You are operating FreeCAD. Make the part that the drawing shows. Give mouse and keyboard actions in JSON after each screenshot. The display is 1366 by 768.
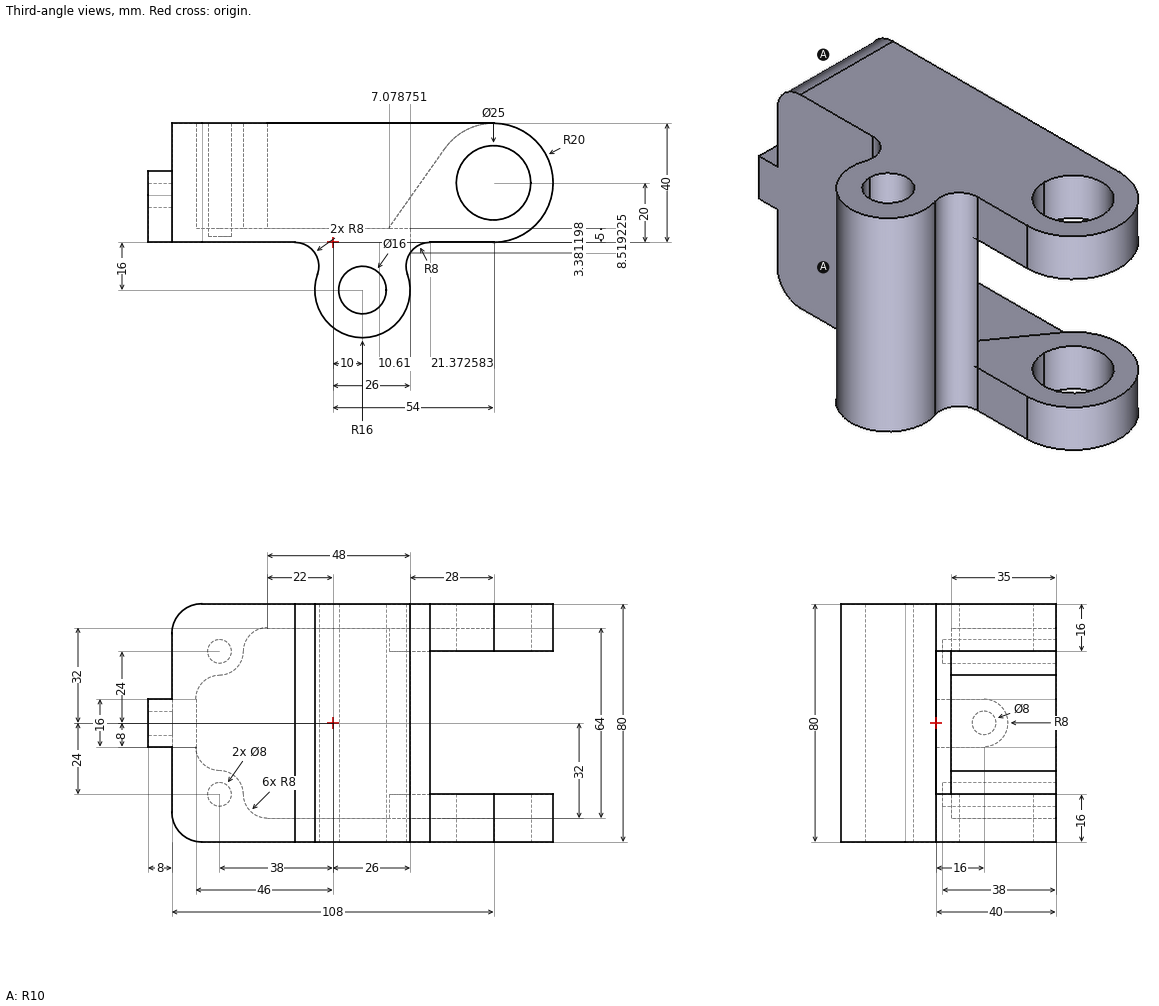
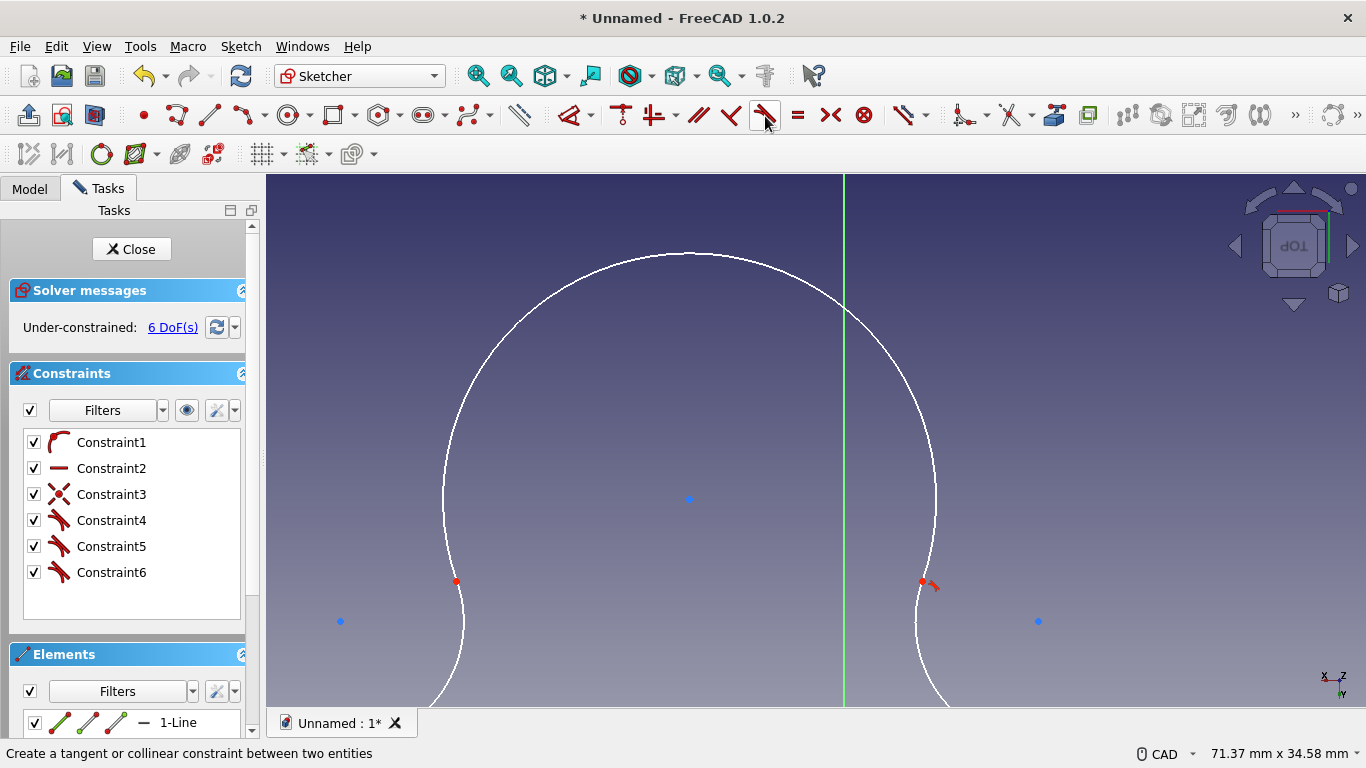
{"action": "left_click", "coordinate": [860, 322]}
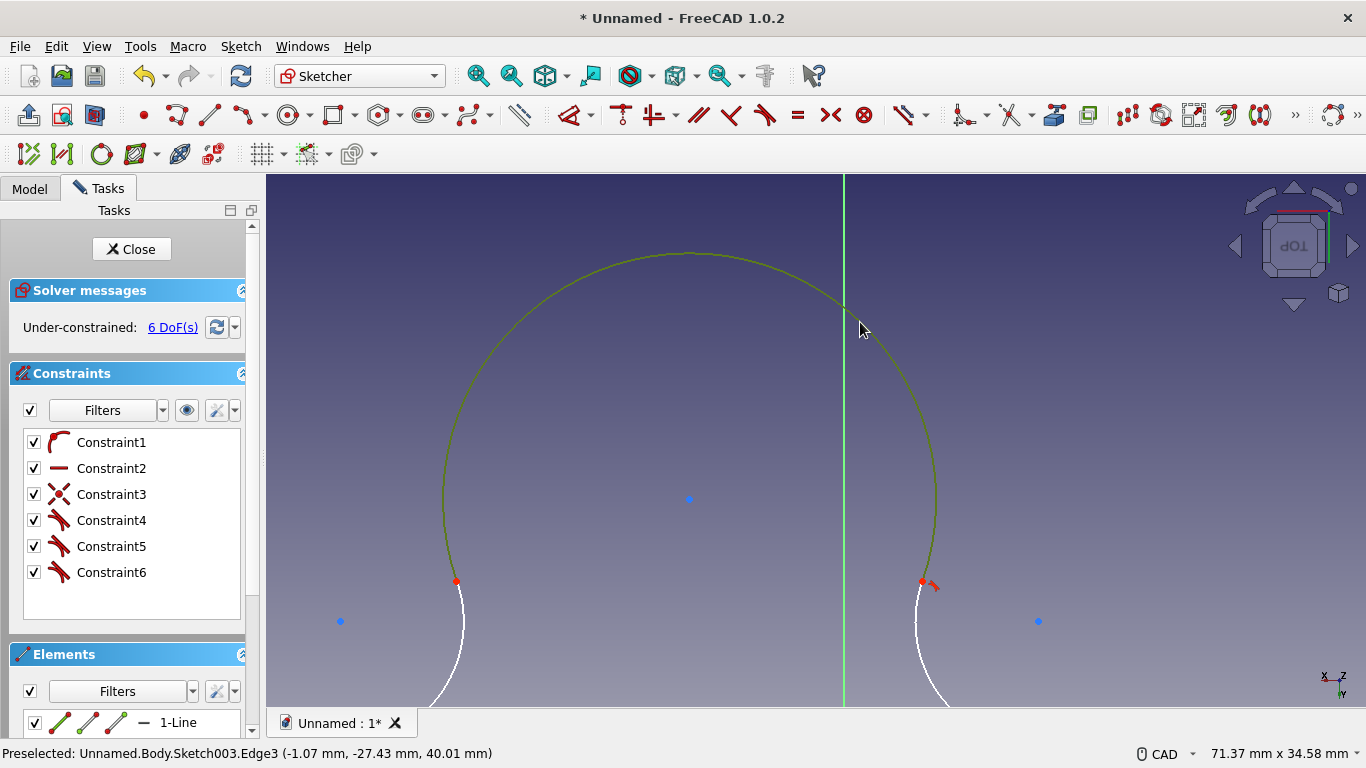
{"action": "left_click", "coordinate": [460, 651]}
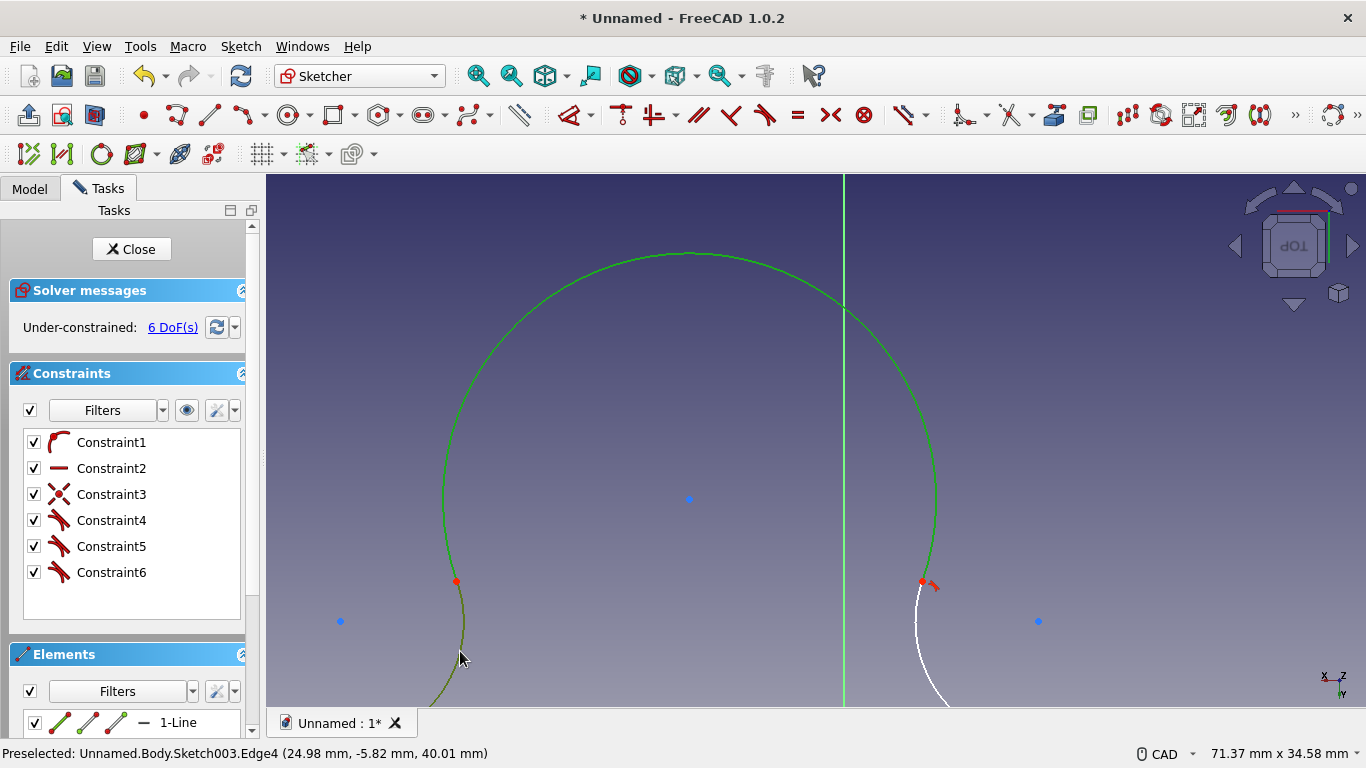
{"action": "left_click", "coordinate": [765, 116]}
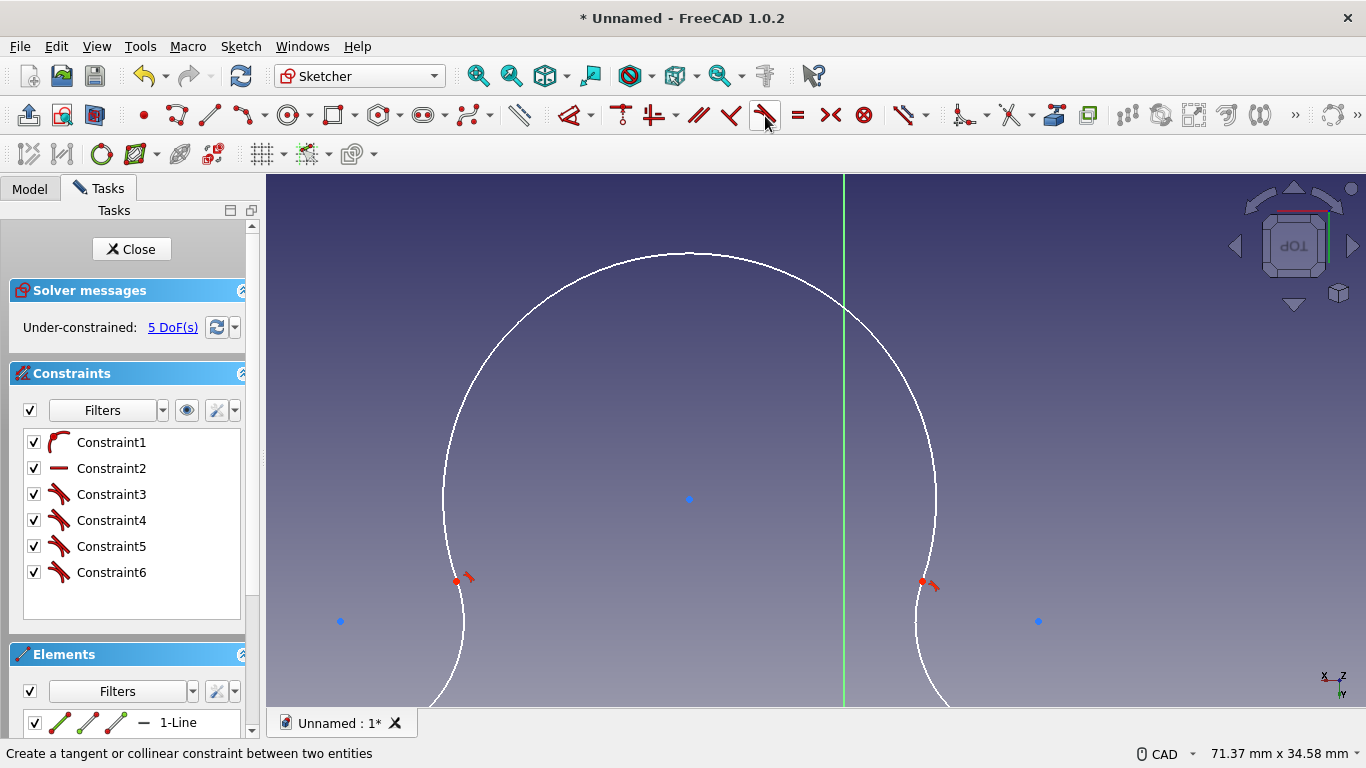
{"action": "left_click", "coordinate": [919, 651]}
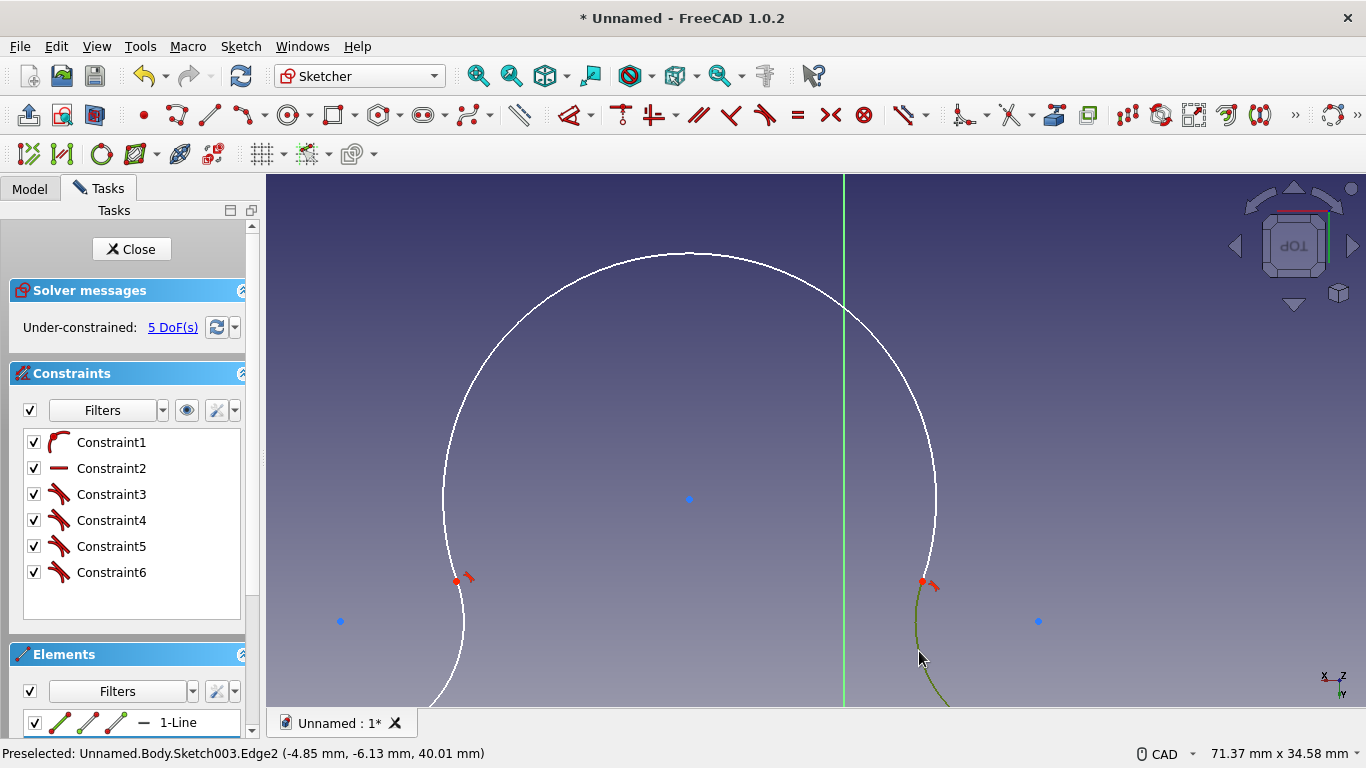
{"action": "left_click", "coordinate": [460, 651]}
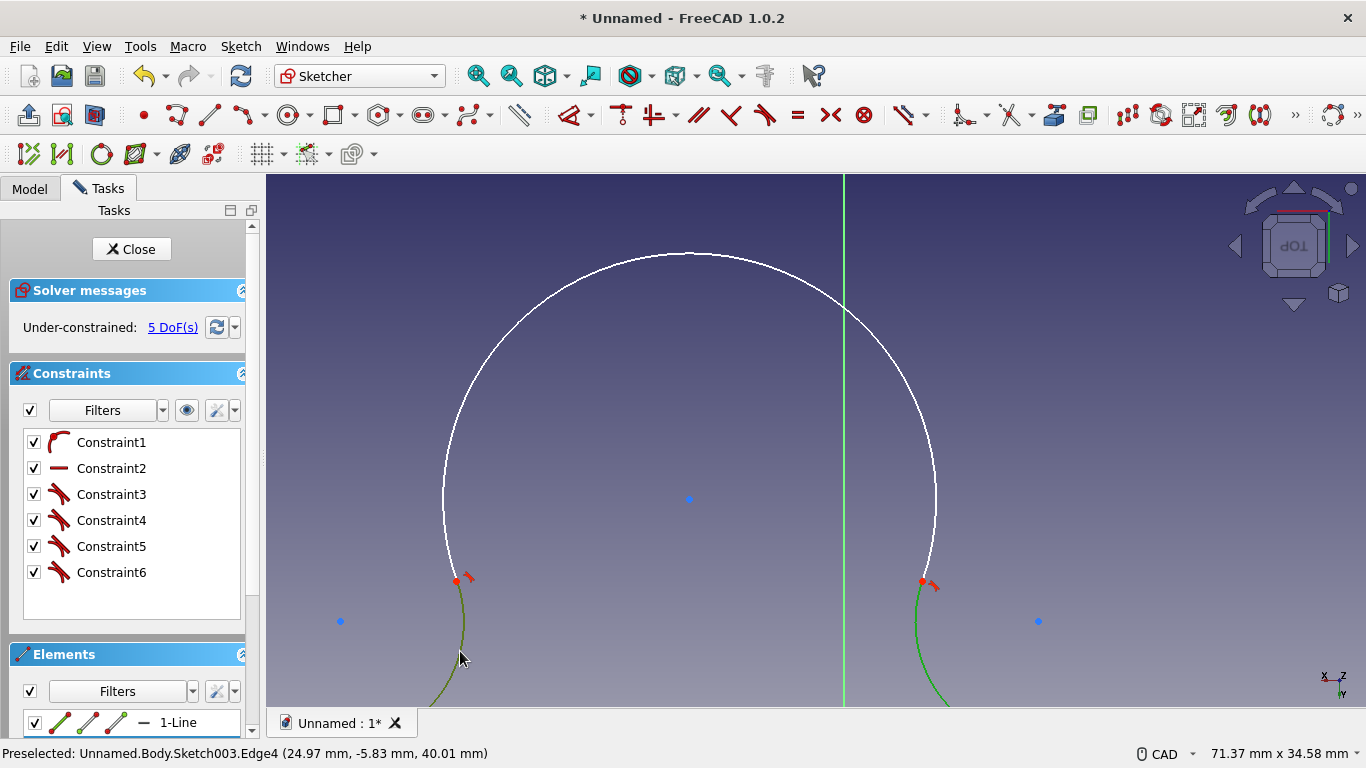
{"action": "key", "text": "e"}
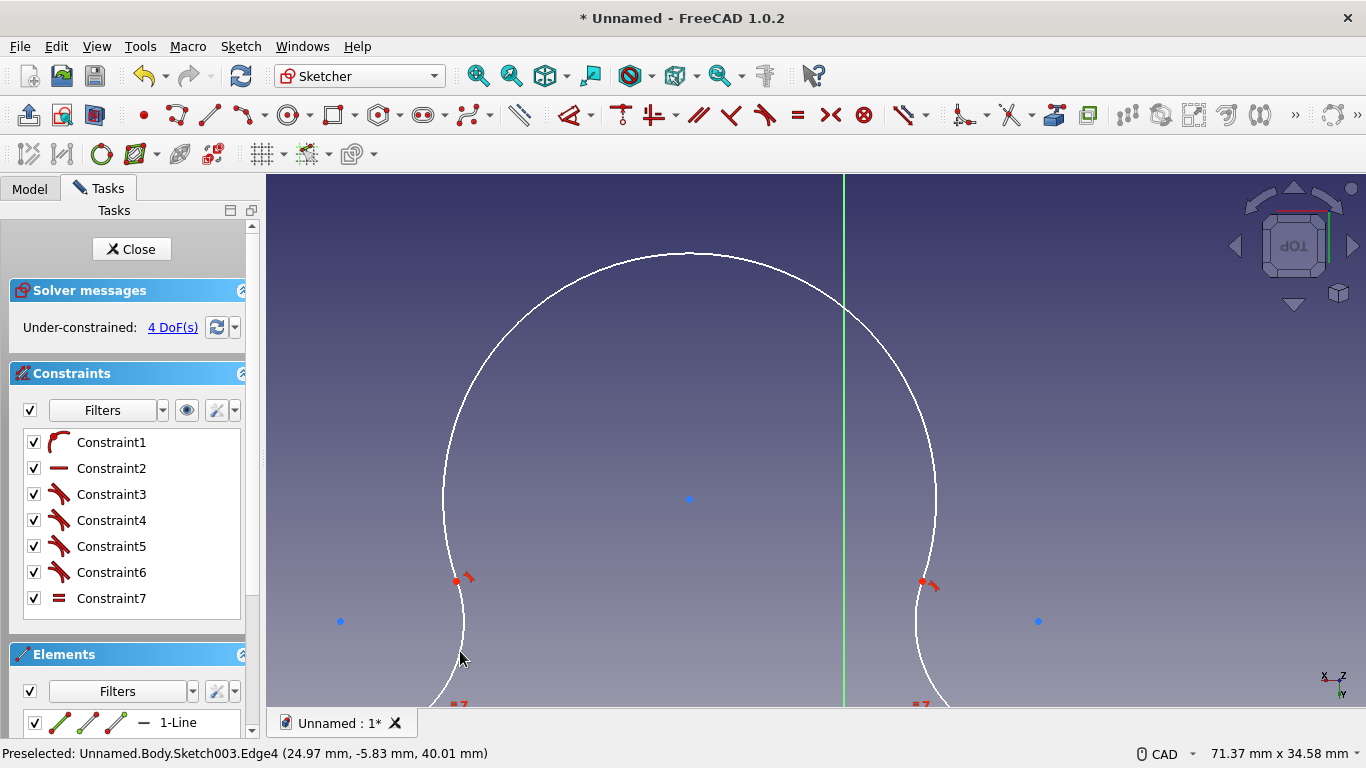
{"action": "left_click", "coordinate": [568, 116]}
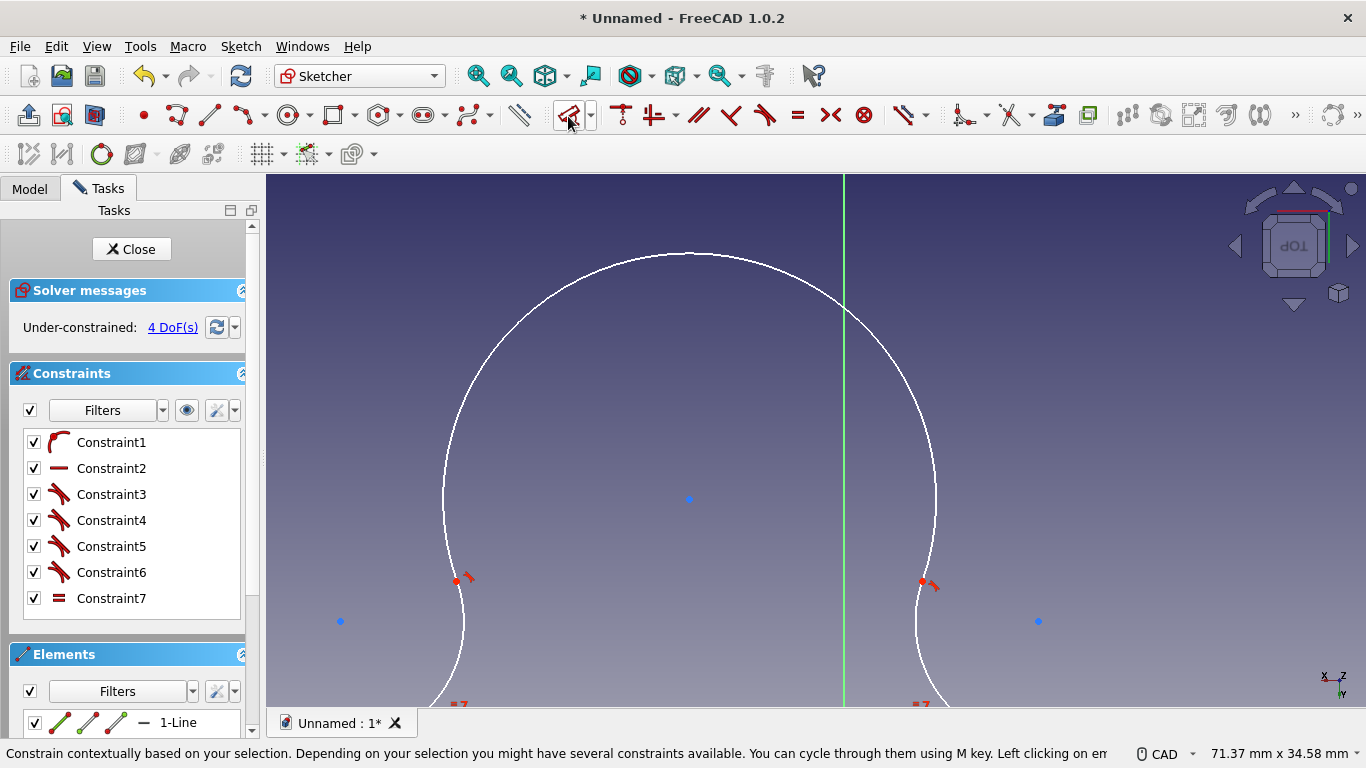
{"action": "left_click", "coordinate": [919, 651]}
{"action": "left_click", "coordinate": [888, 659]}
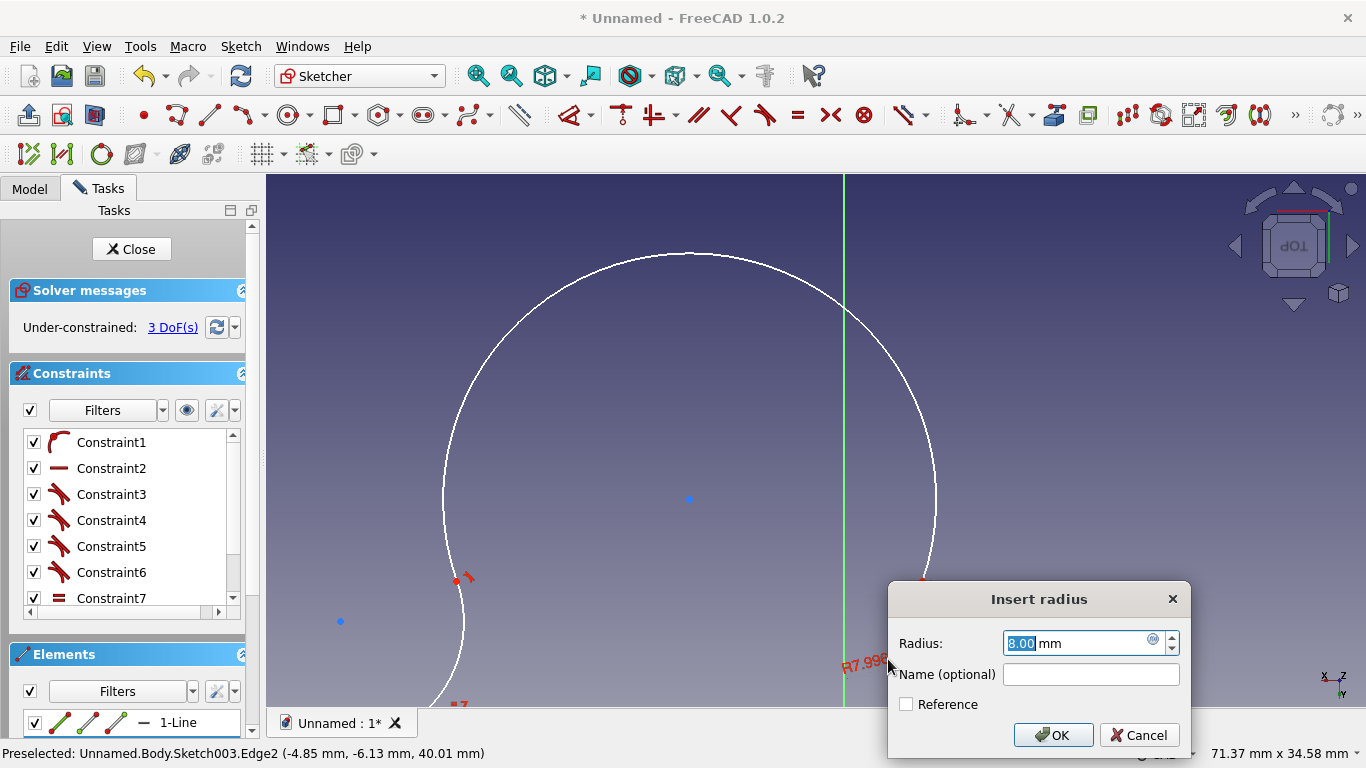
{"action": "type", "text": "8"}
{"action": "key", "text": "Return"}